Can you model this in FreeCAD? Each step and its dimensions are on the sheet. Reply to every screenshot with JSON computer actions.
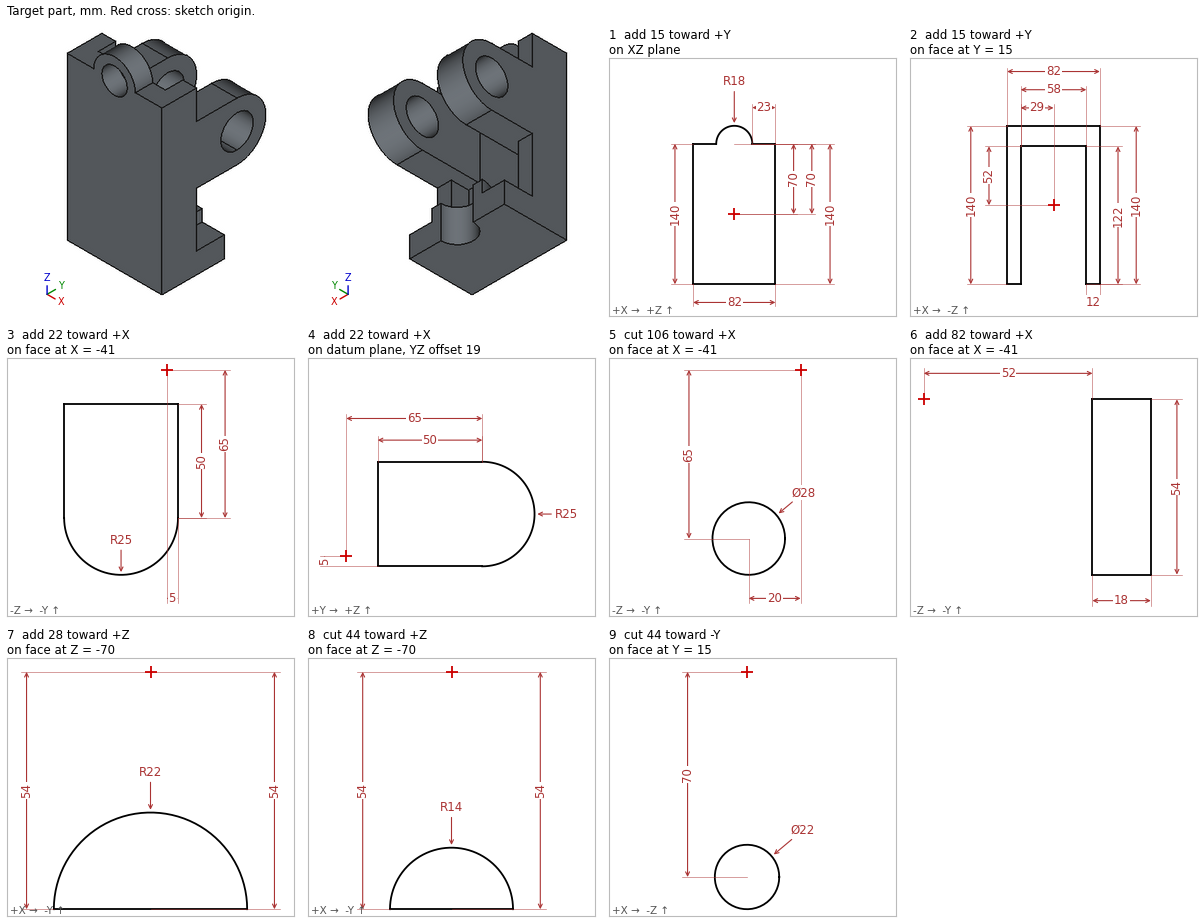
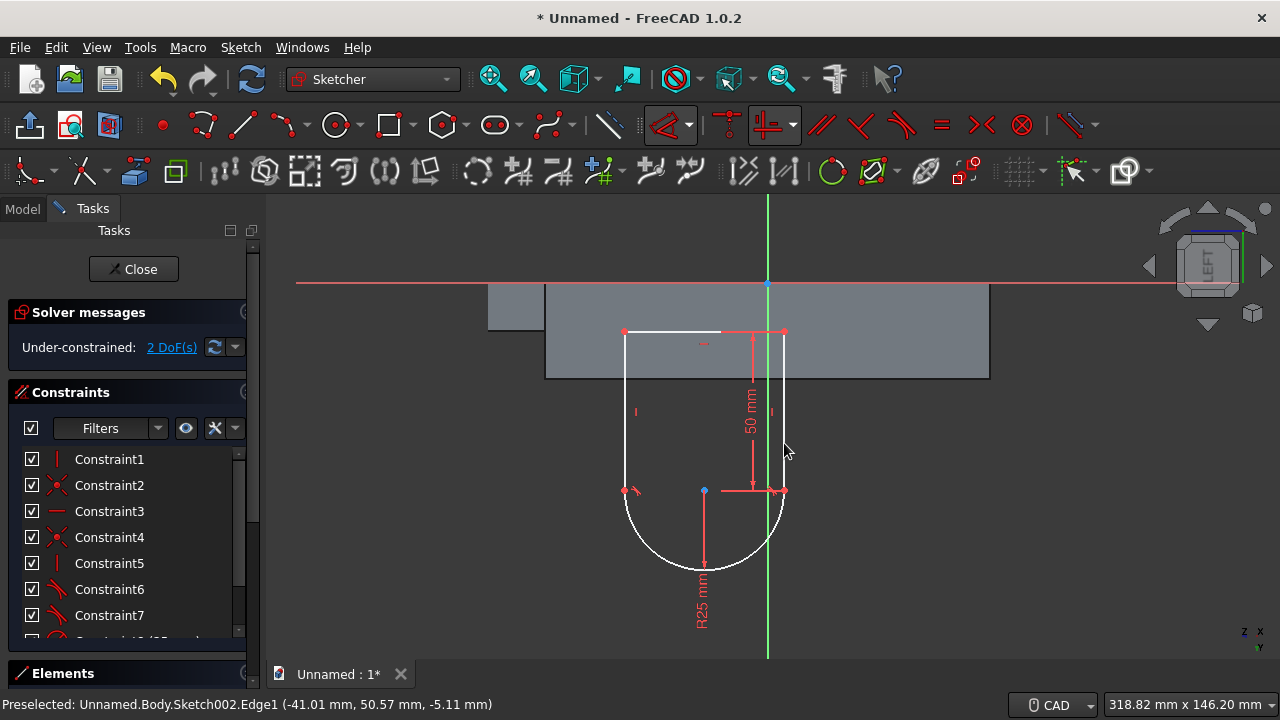
{"action": "scroll", "coordinate": [784, 491], "scroll_direction": "up", "scroll_amount": 5}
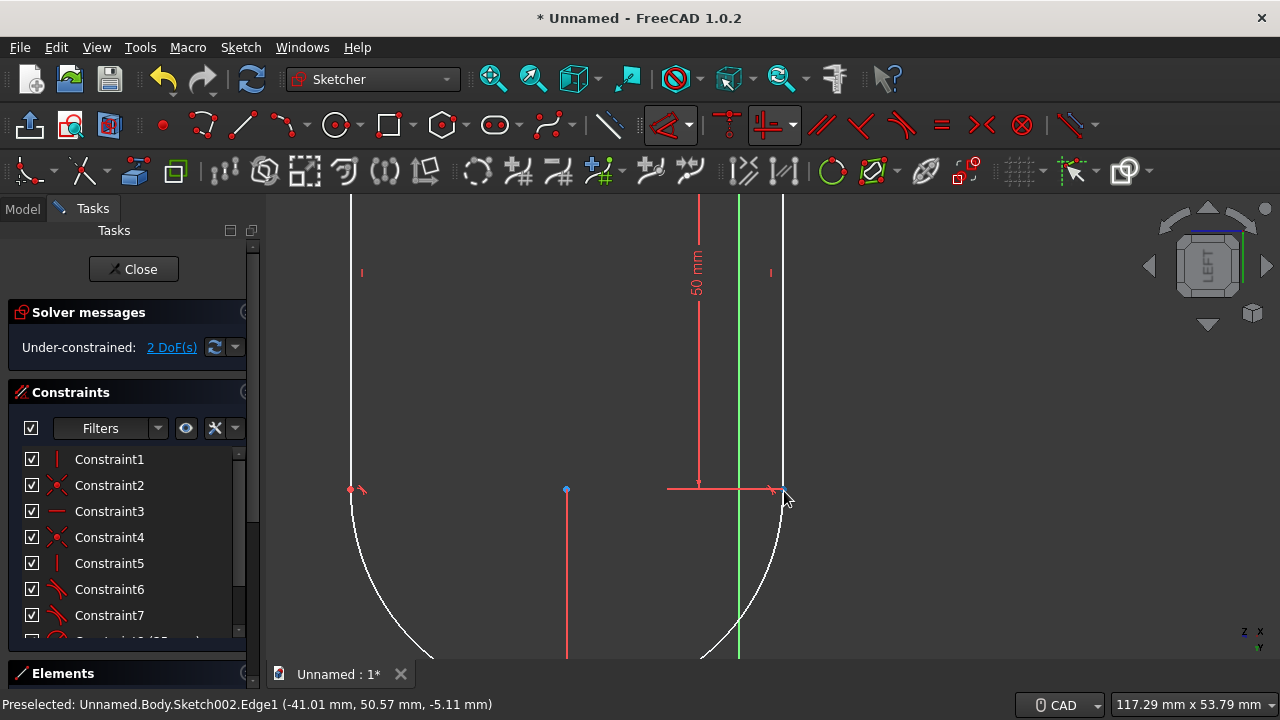
{"action": "left_click", "coordinate": [783, 489]}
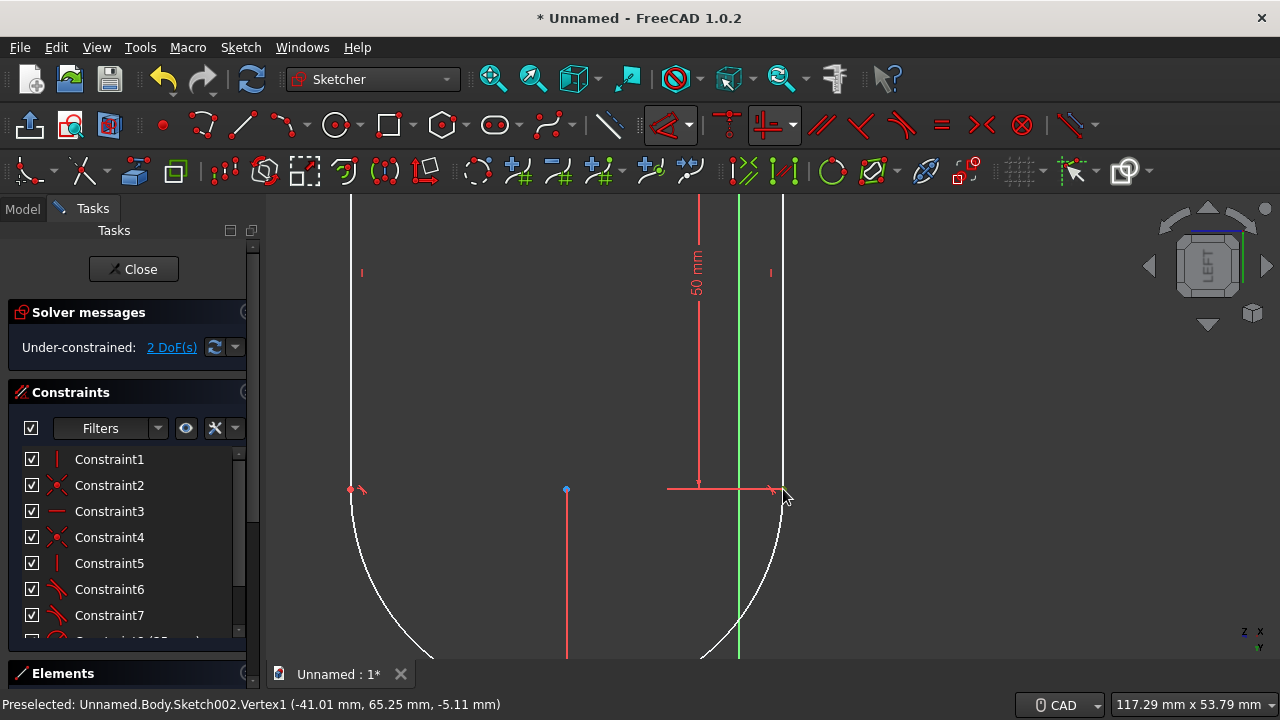
{"action": "key", "text": "l"}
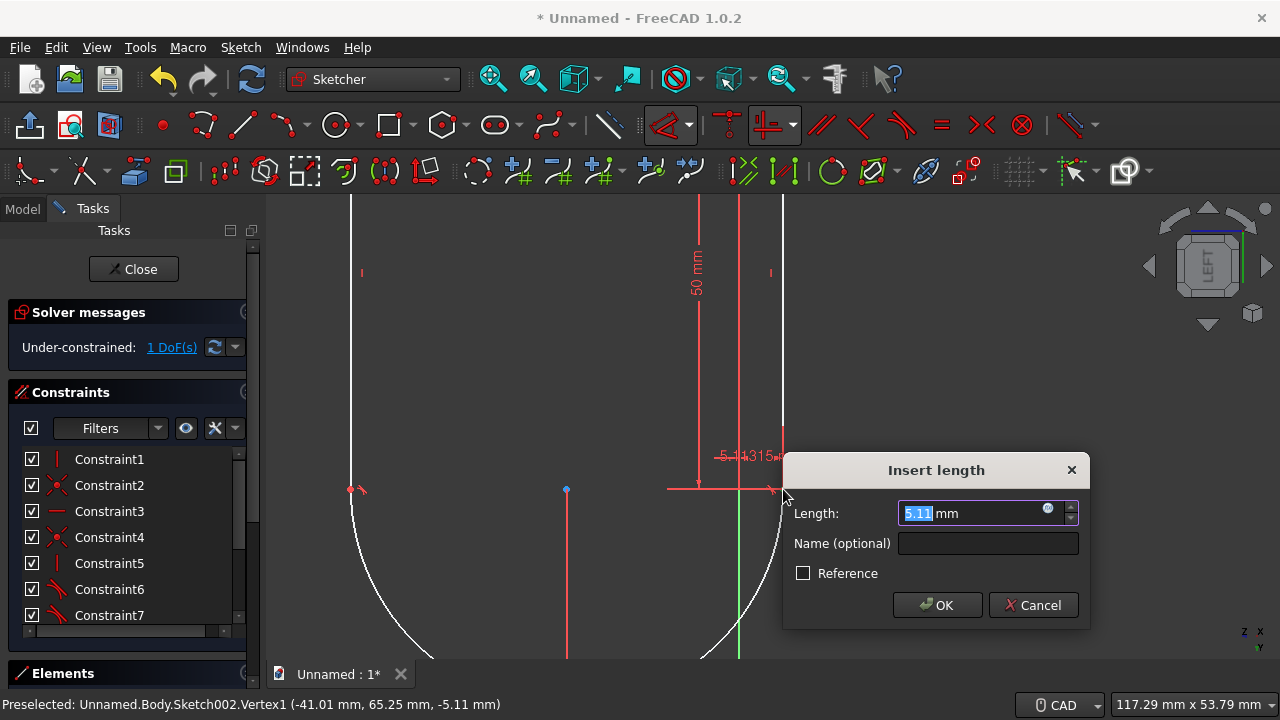
{"action": "type", "text": "5"}
{"action": "key", "text": "Return"}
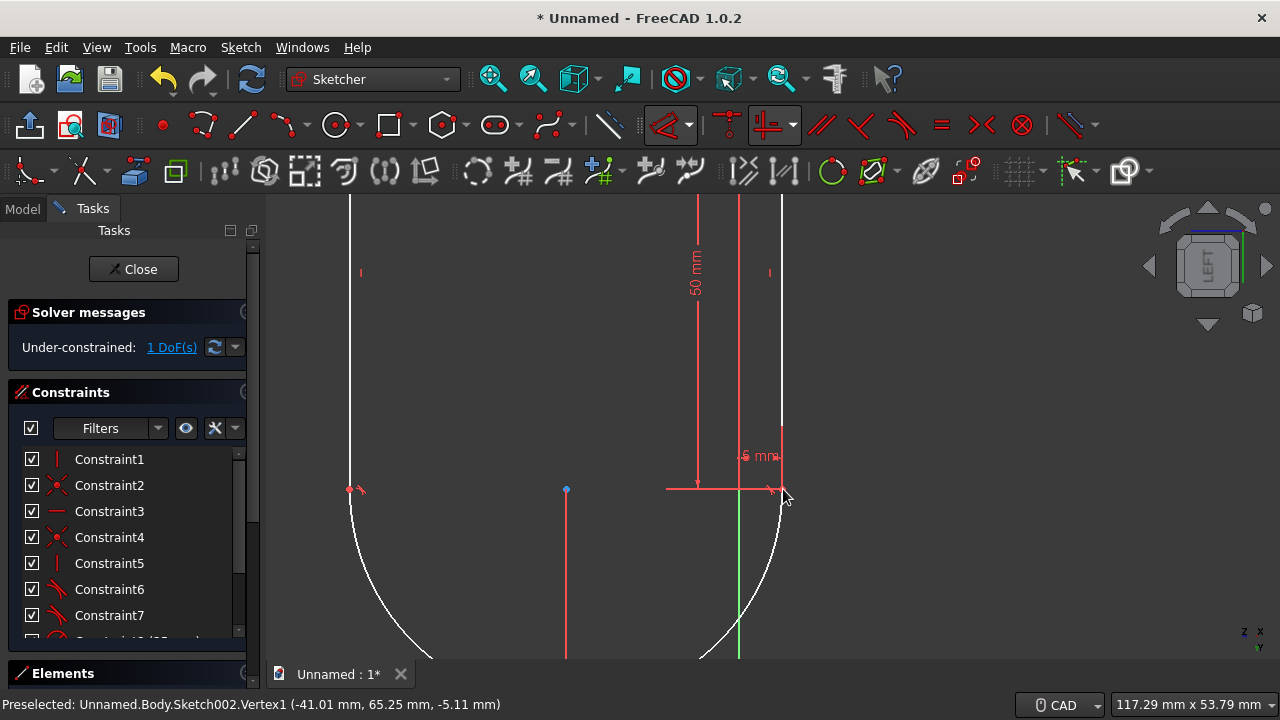
{"action": "left_click", "coordinate": [782, 489]}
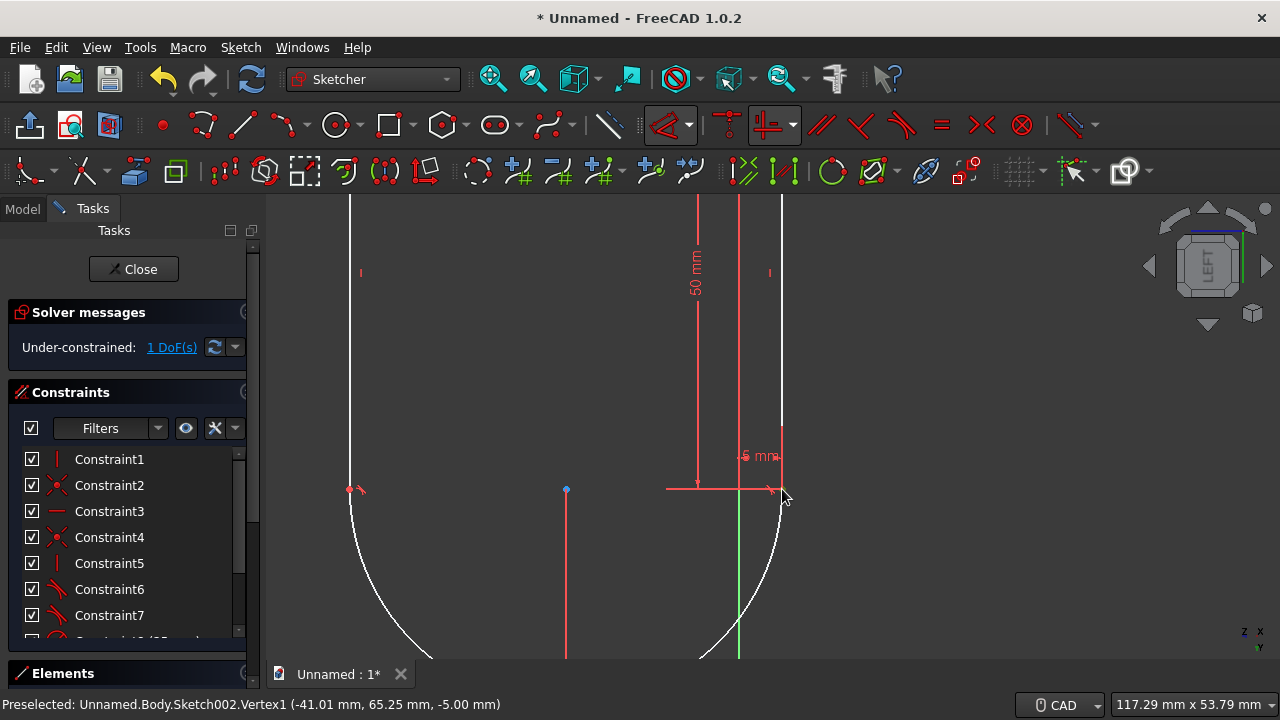
{"action": "key", "text": "i"}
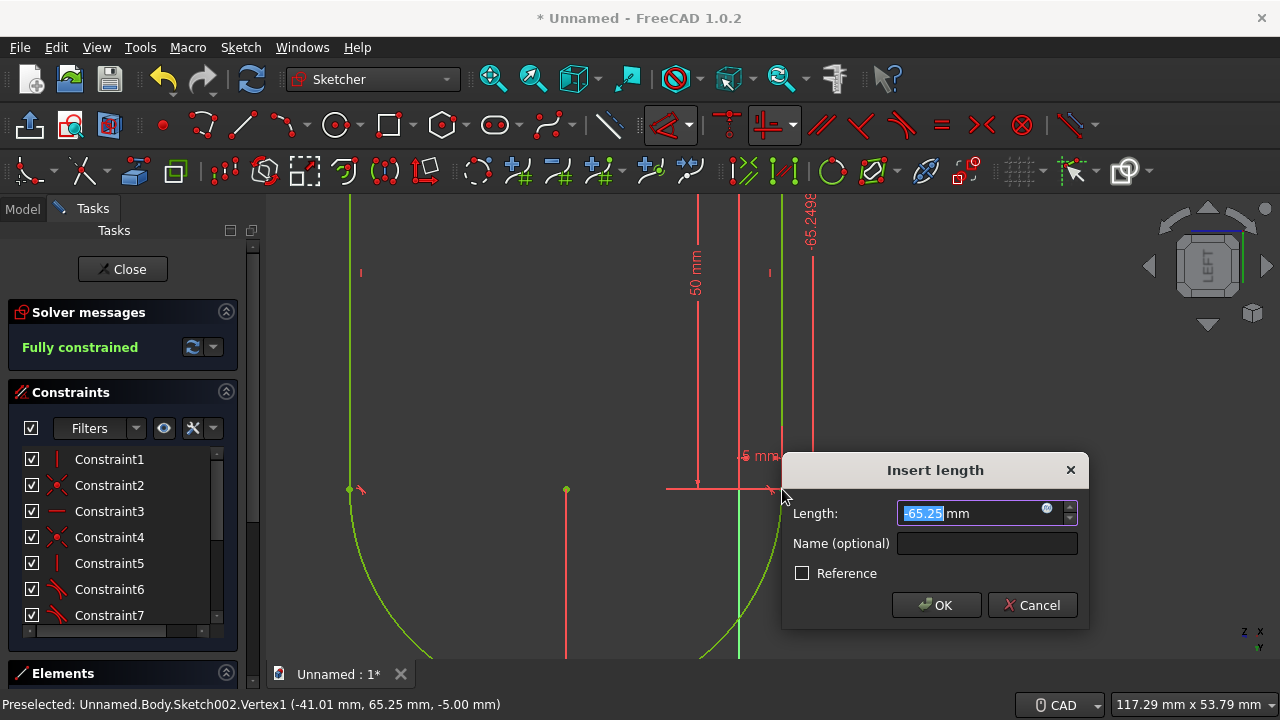
{"action": "type", "text": "-65"}
{"action": "key", "text": "Return"}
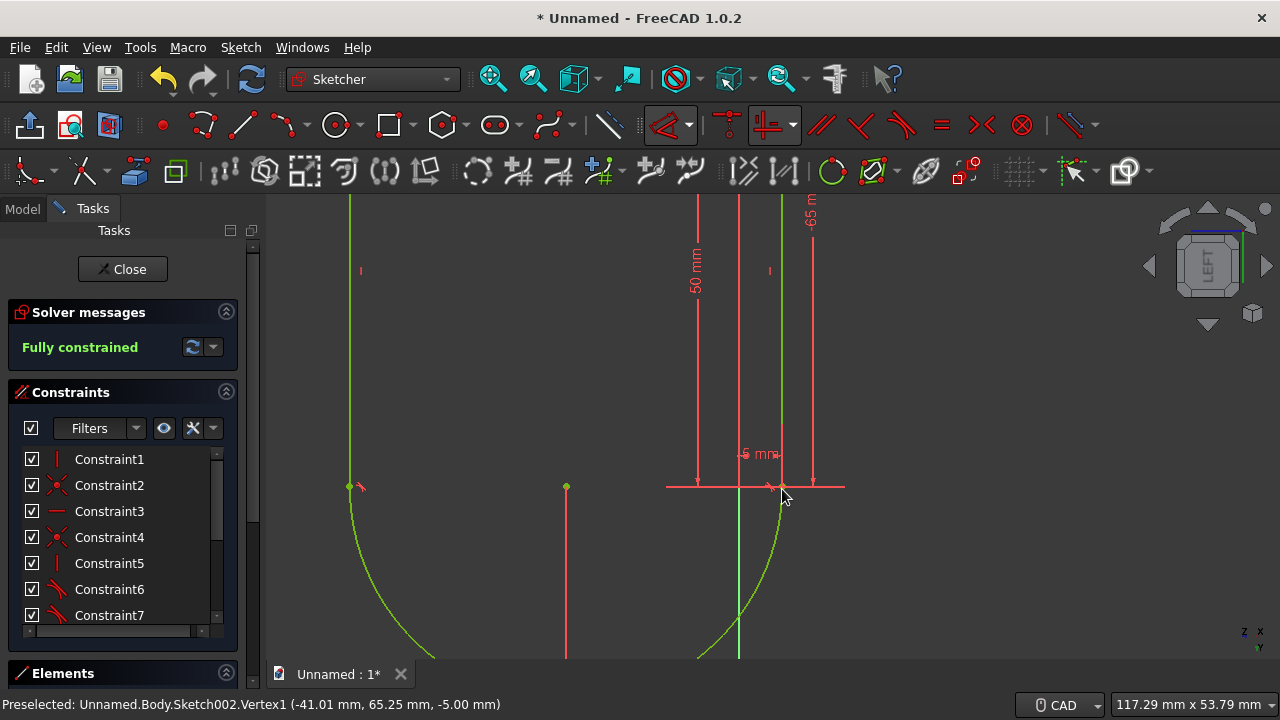
{"action": "left_click", "coordinate": [123, 269]}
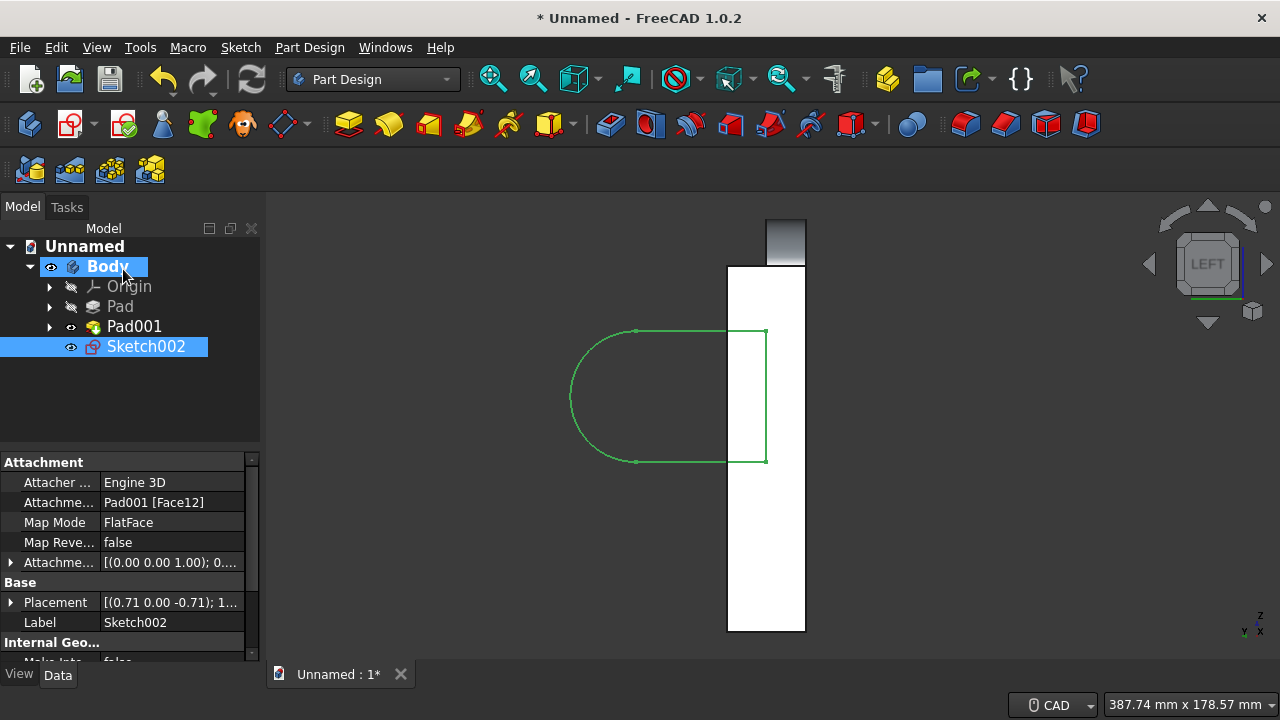
{"action": "left_click", "coordinate": [350, 124]}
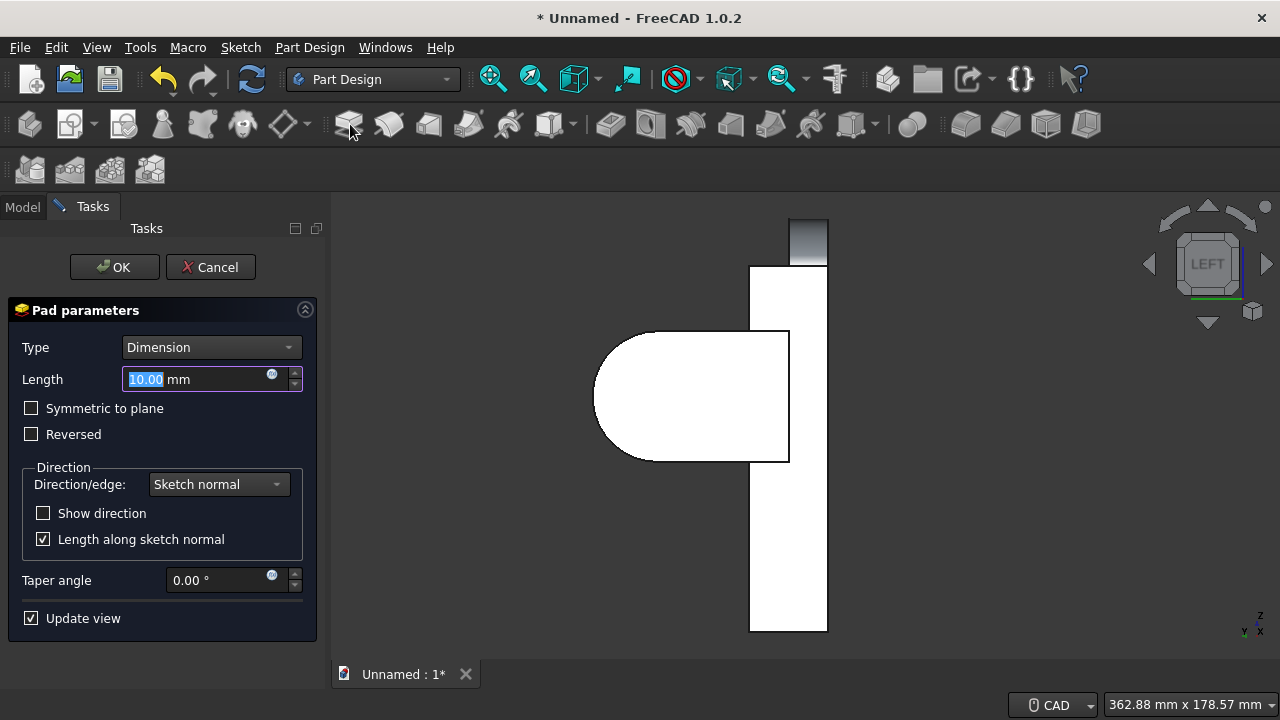
{"action": "type", "text": "22"}
{"action": "key", "text": "Tab"}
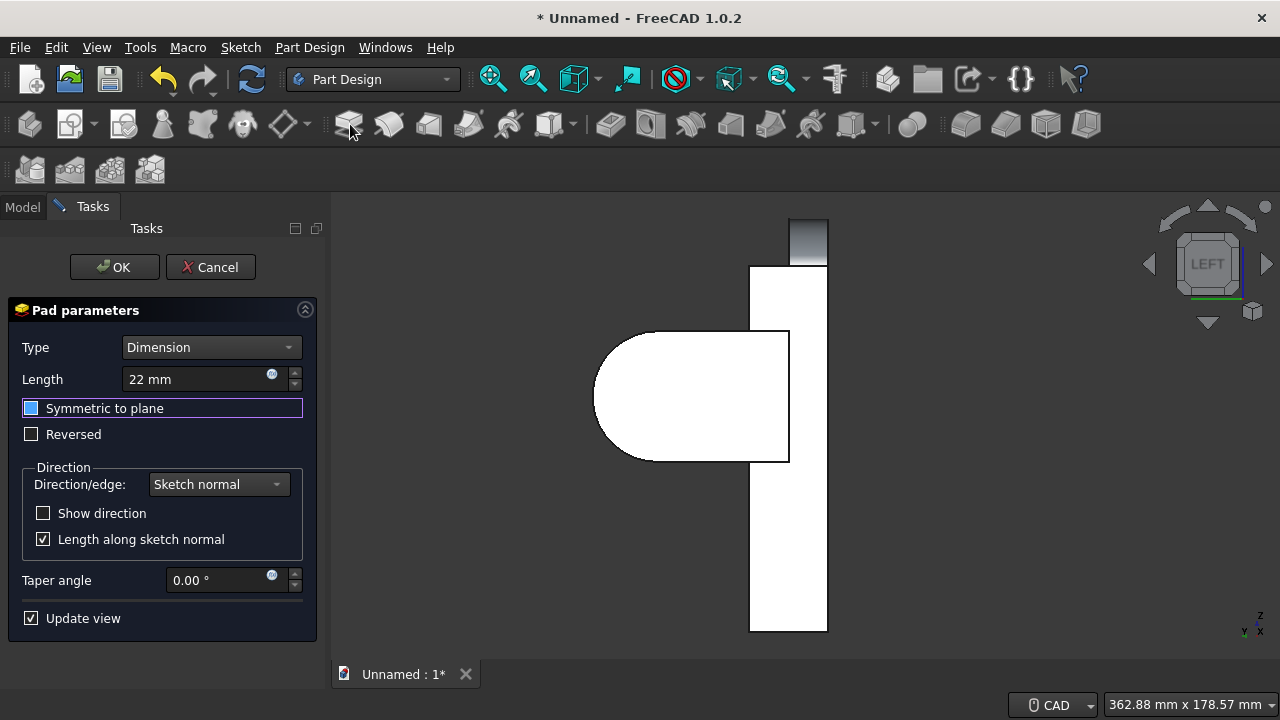
{"action": "left_click", "coordinate": [30, 434]}